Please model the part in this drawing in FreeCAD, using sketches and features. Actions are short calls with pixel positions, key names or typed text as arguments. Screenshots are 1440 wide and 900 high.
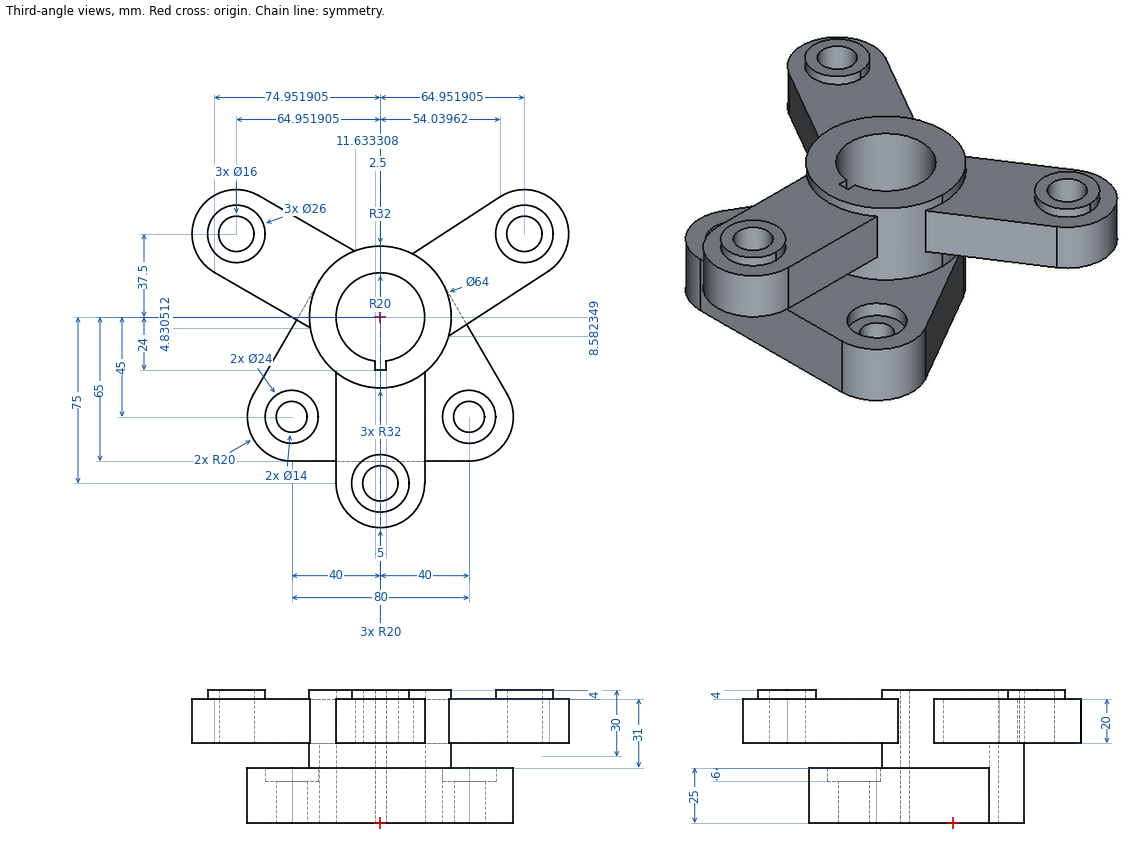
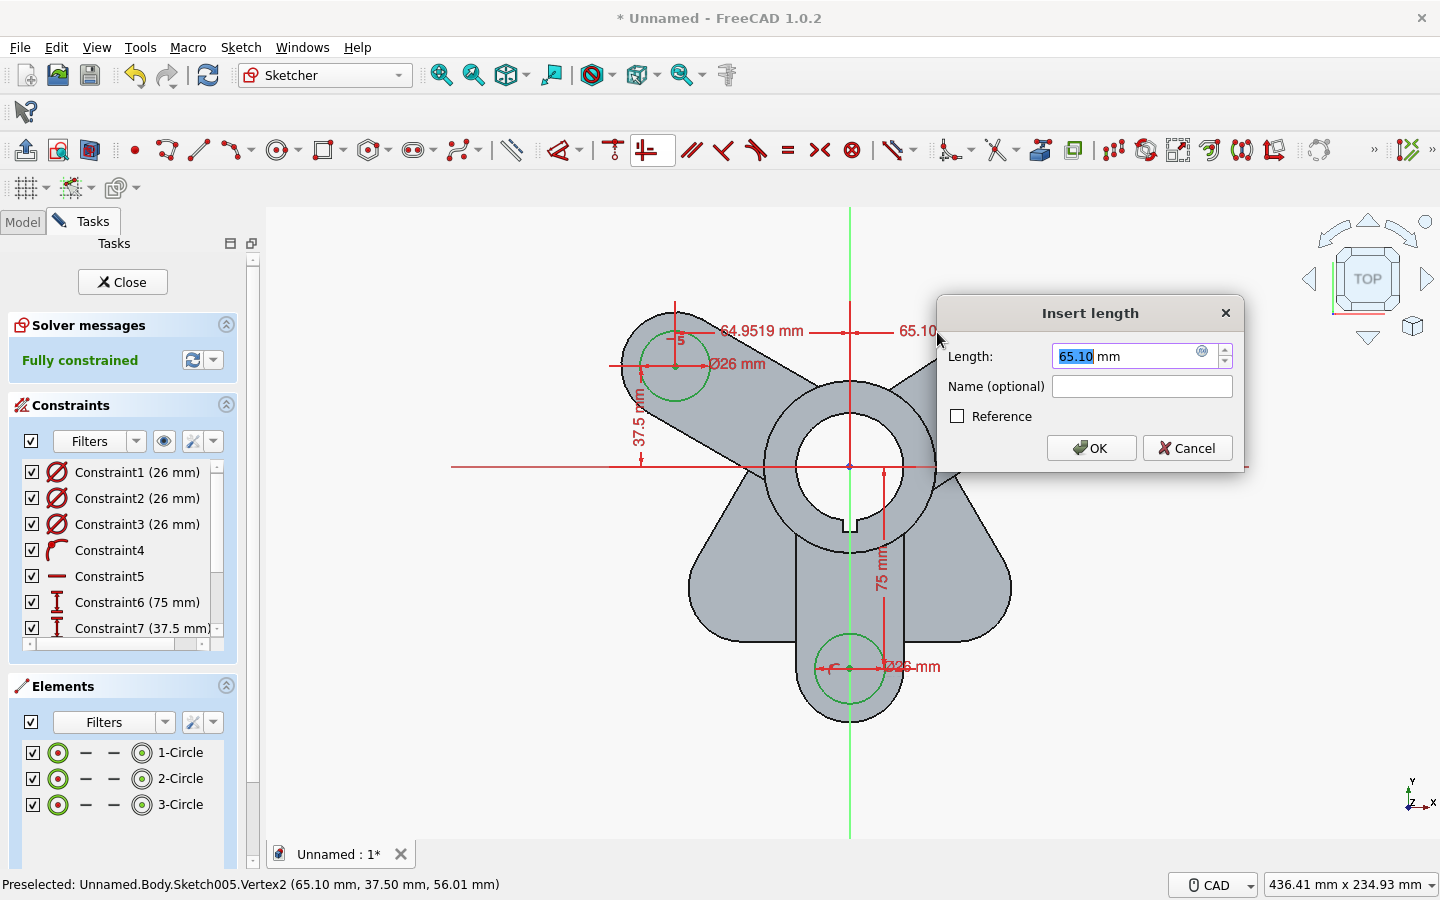
text(64.951905)
key(Return)
key(Escape)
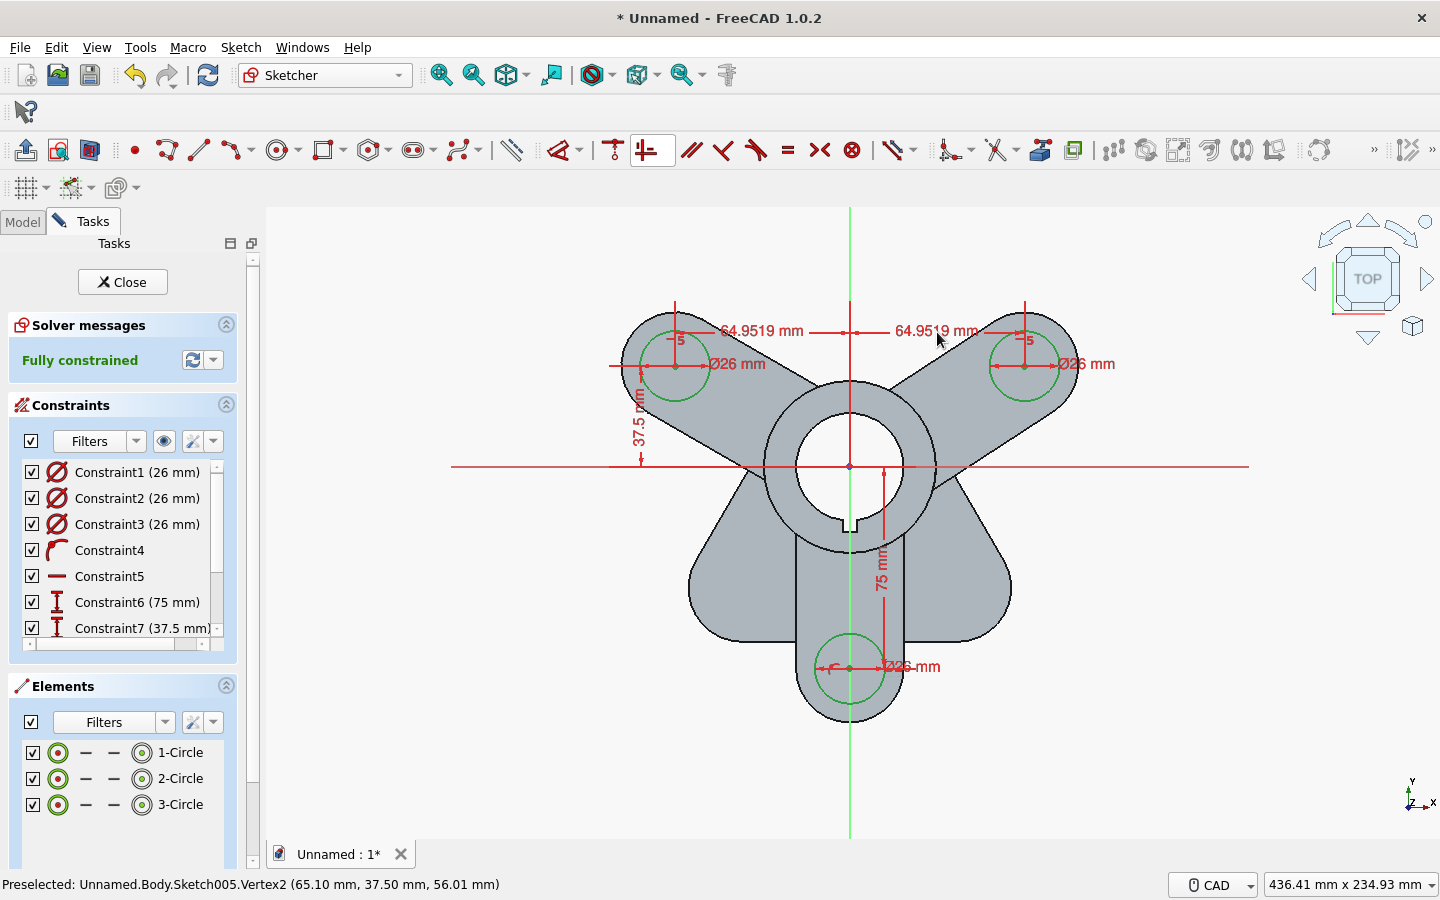
click(123, 282)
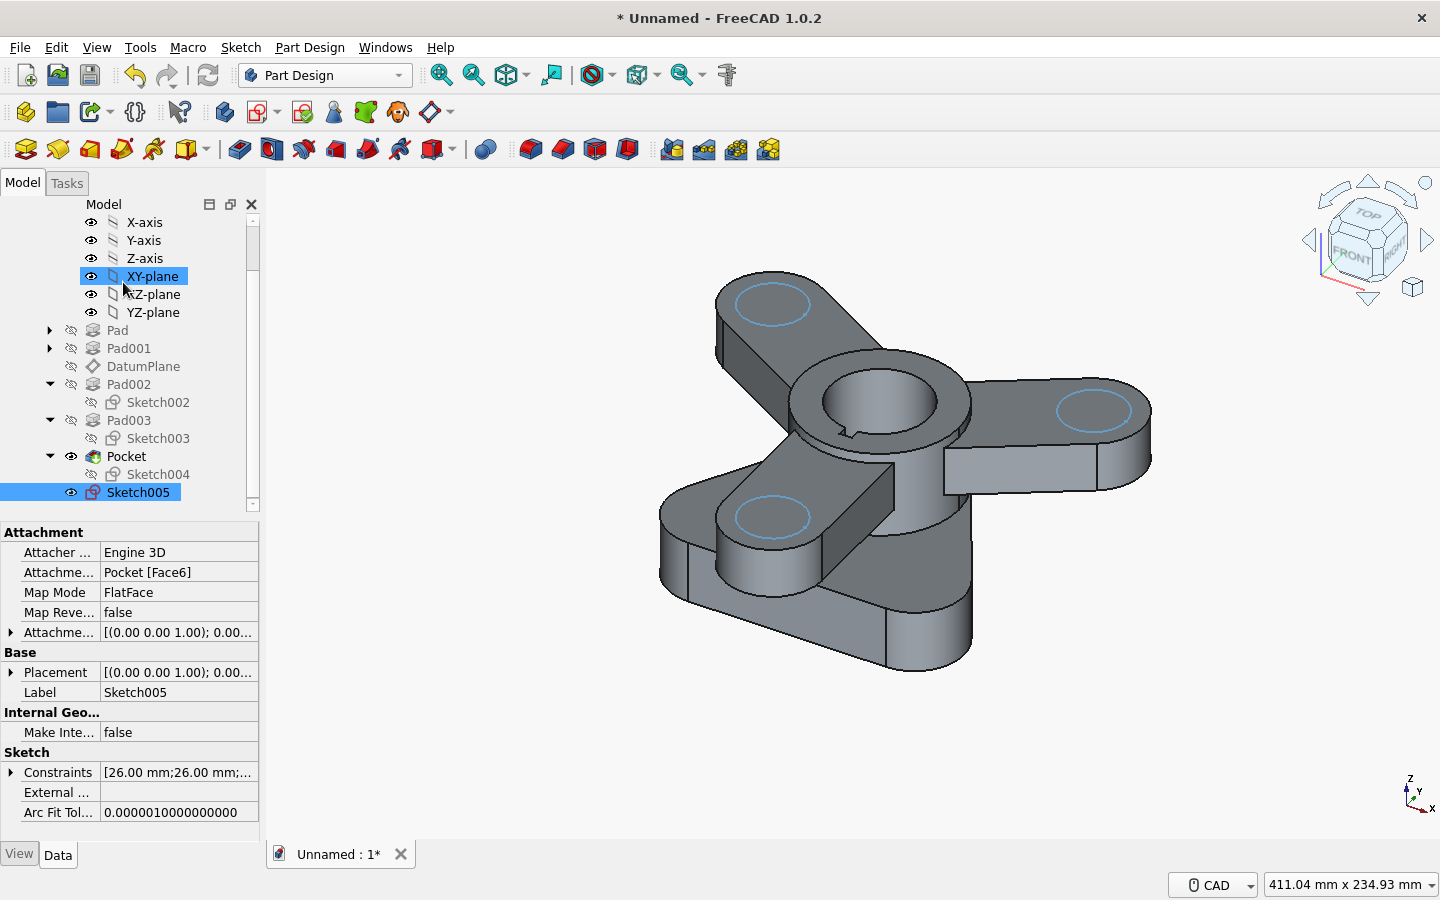
click(26, 150)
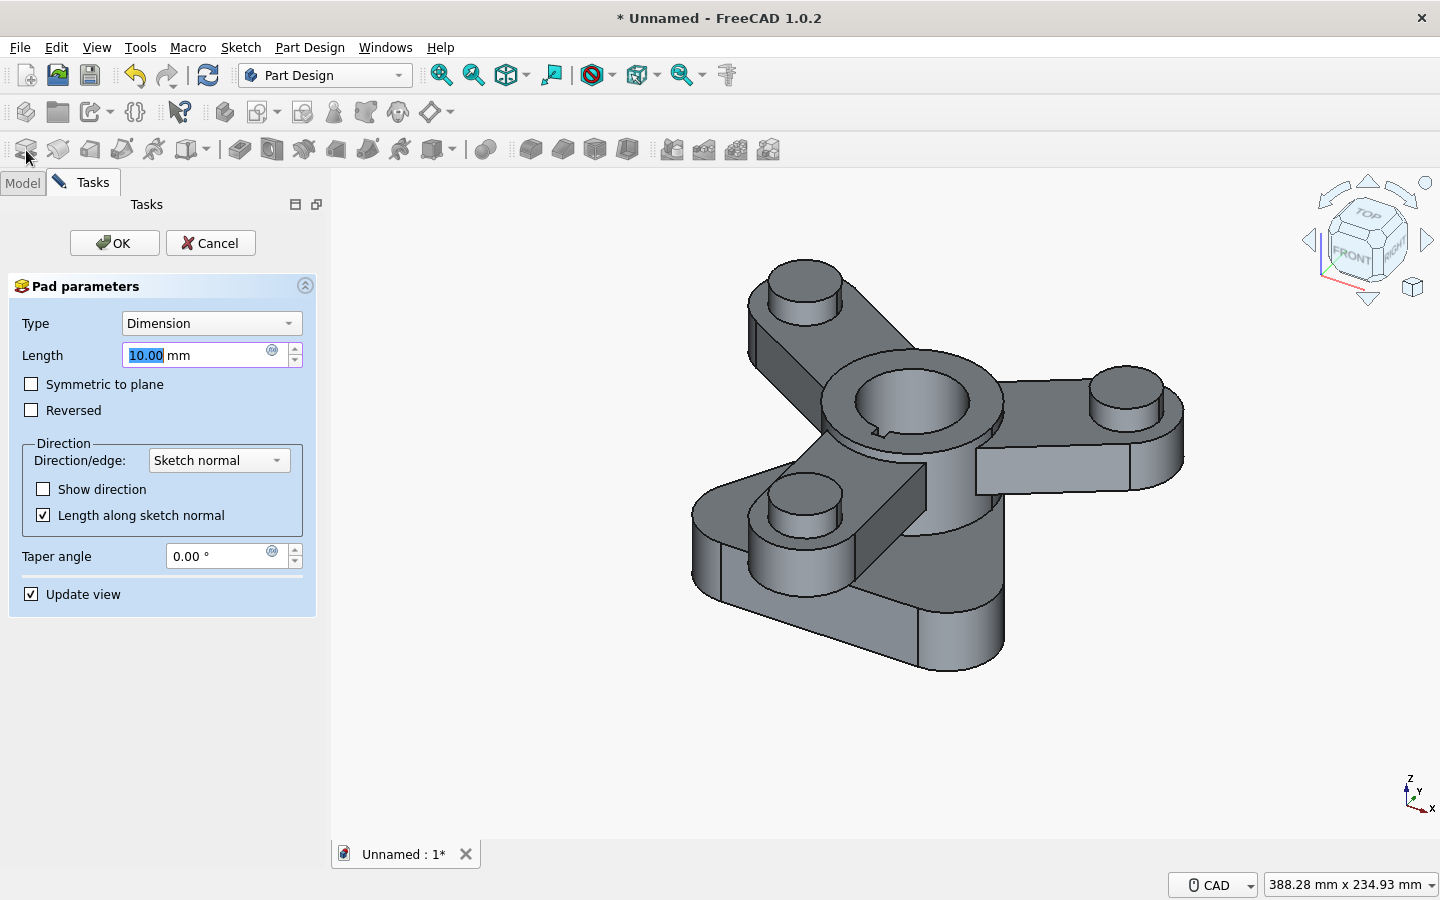
text(4)
key(Tab)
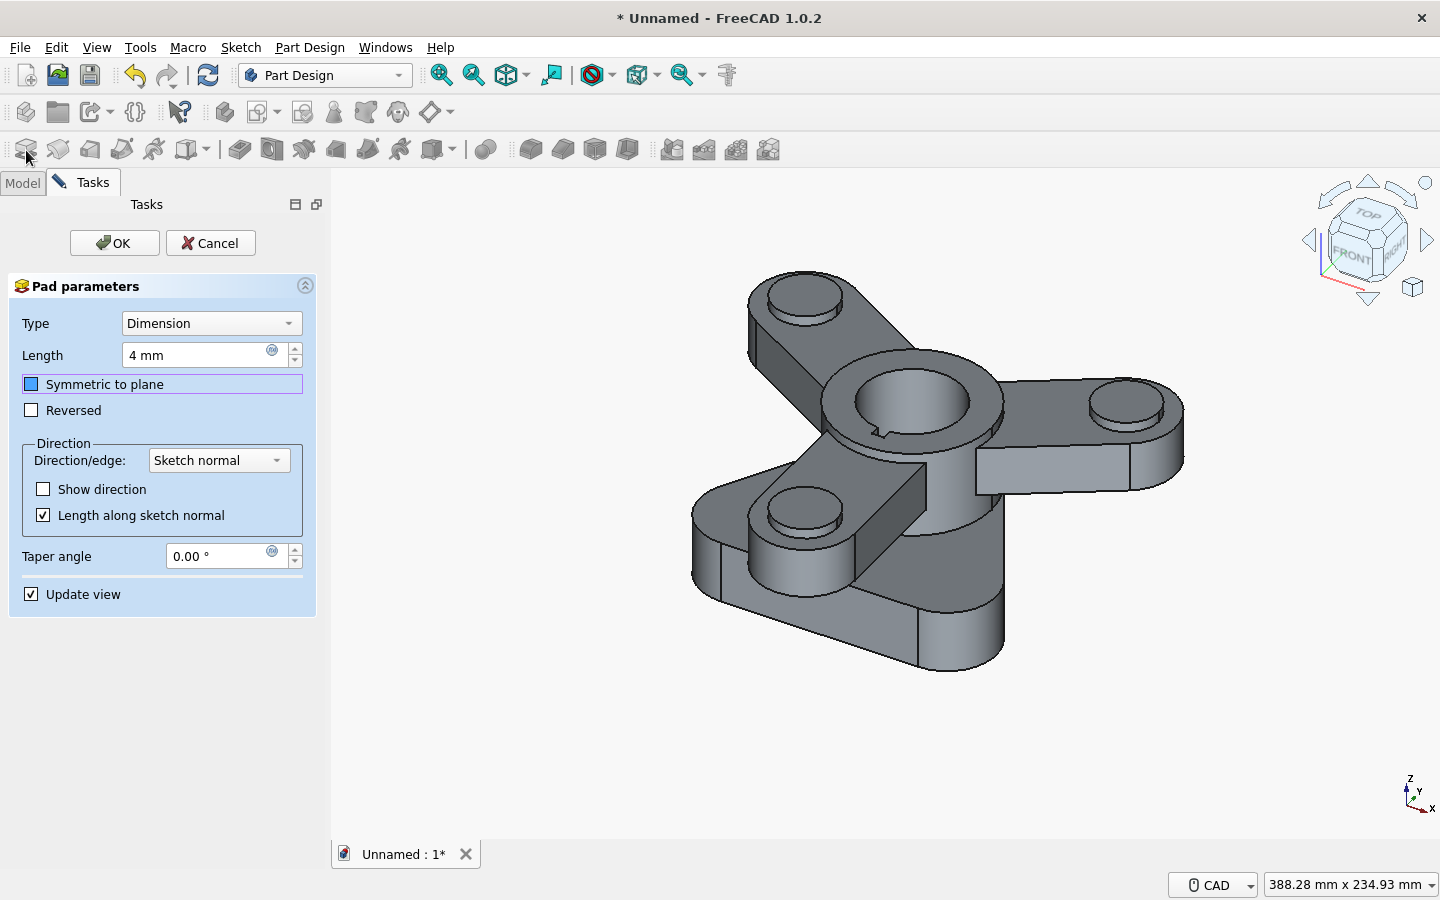
click(115, 243)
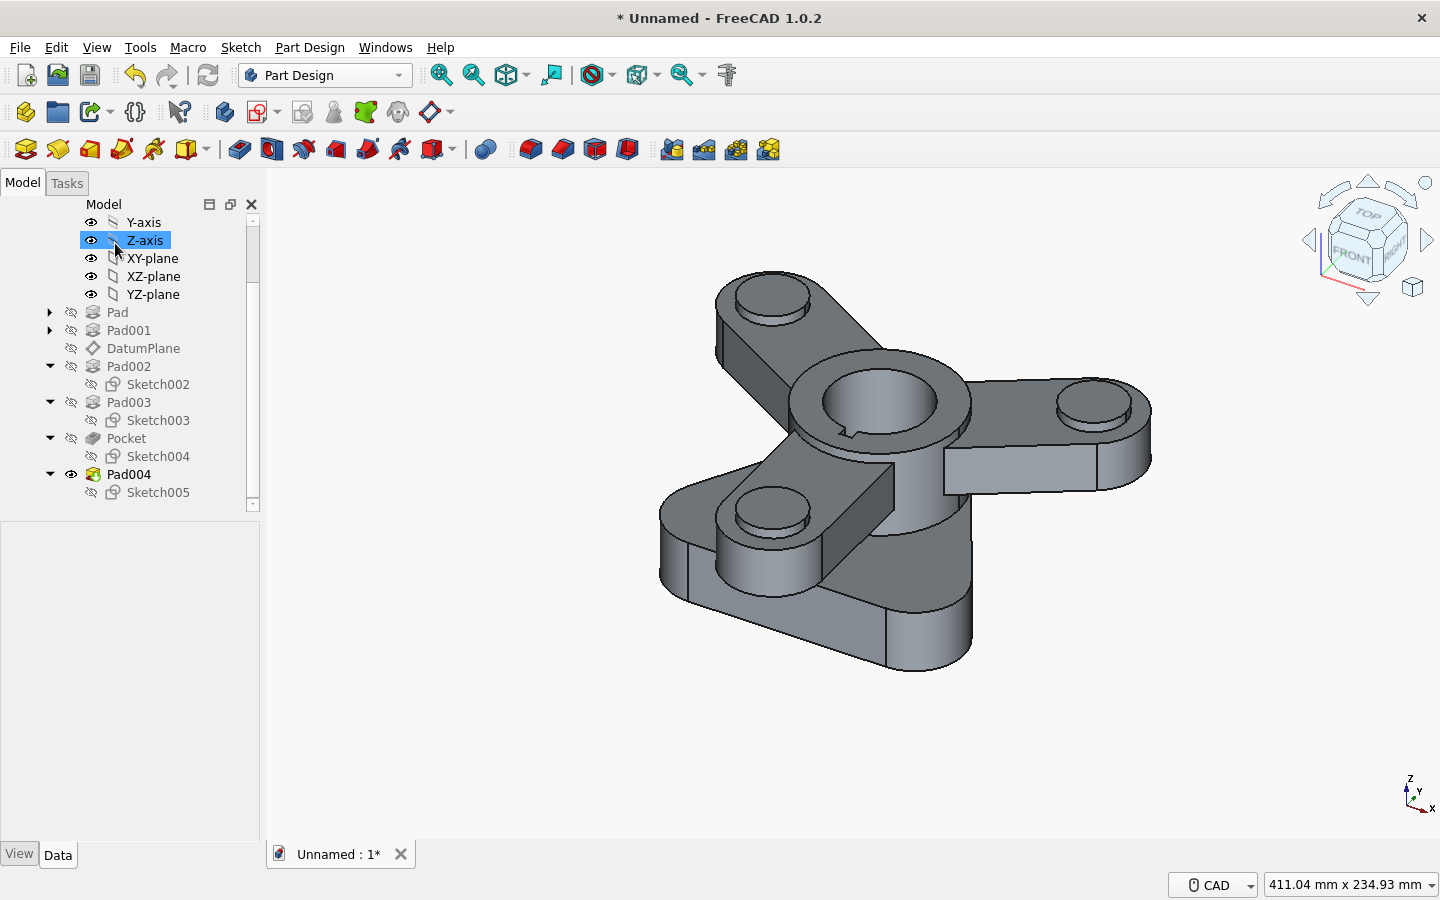
click(861, 360)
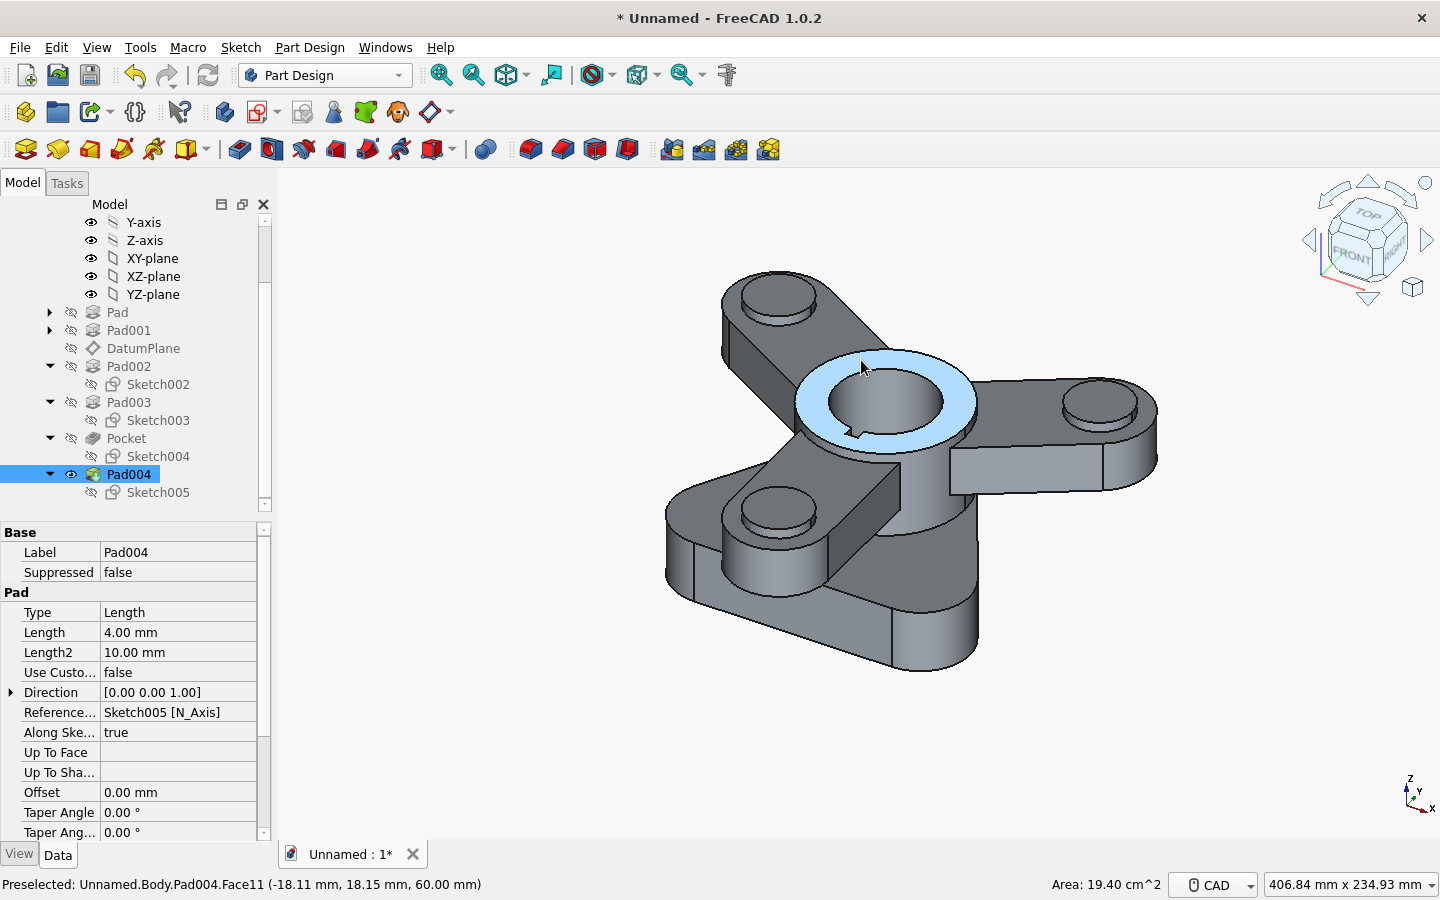
click(258, 112)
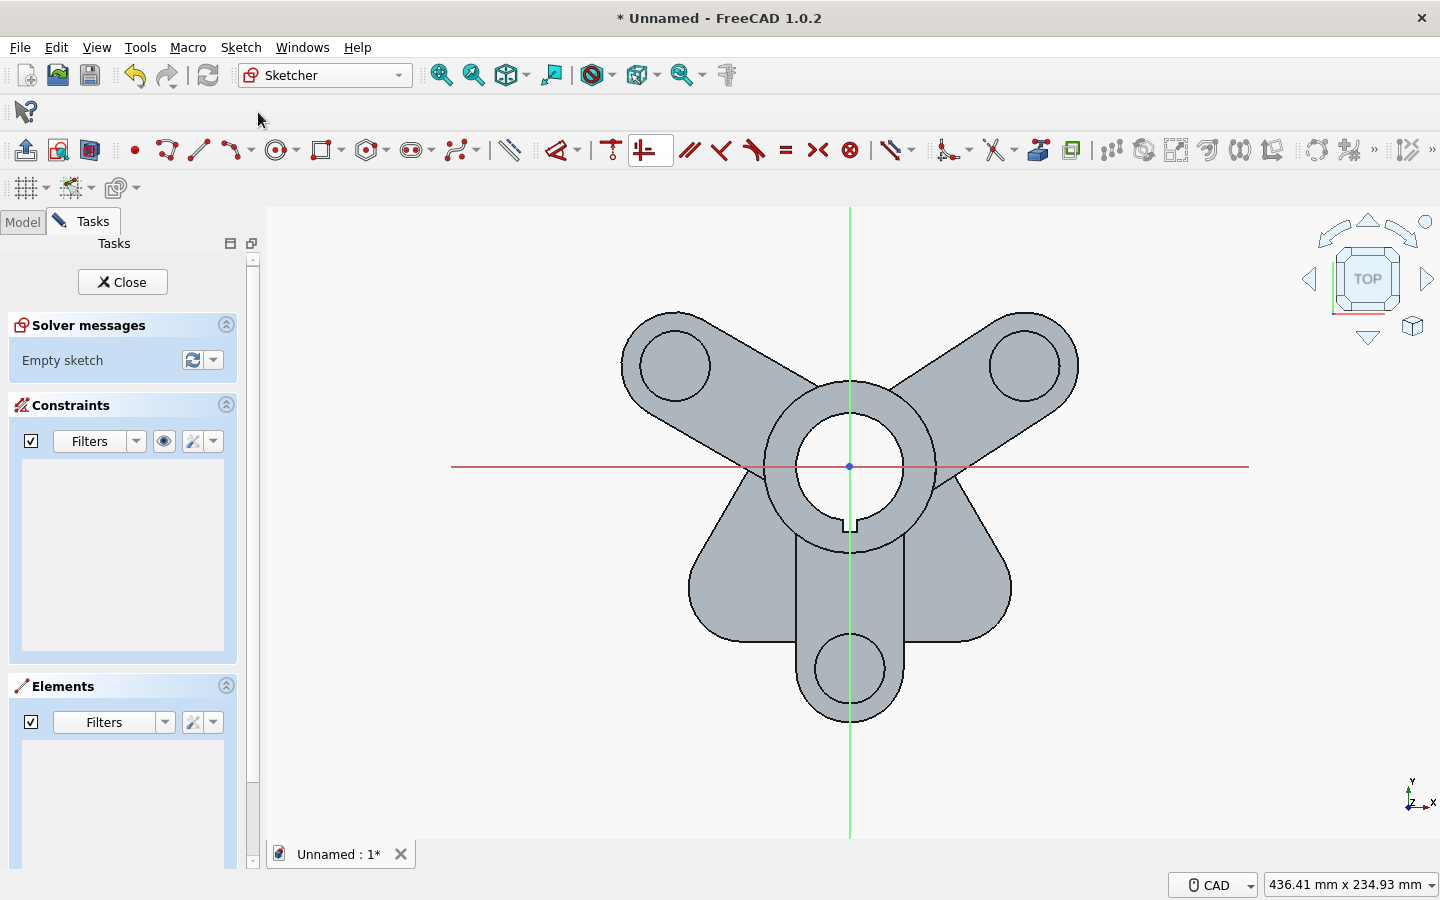
click(276, 150)